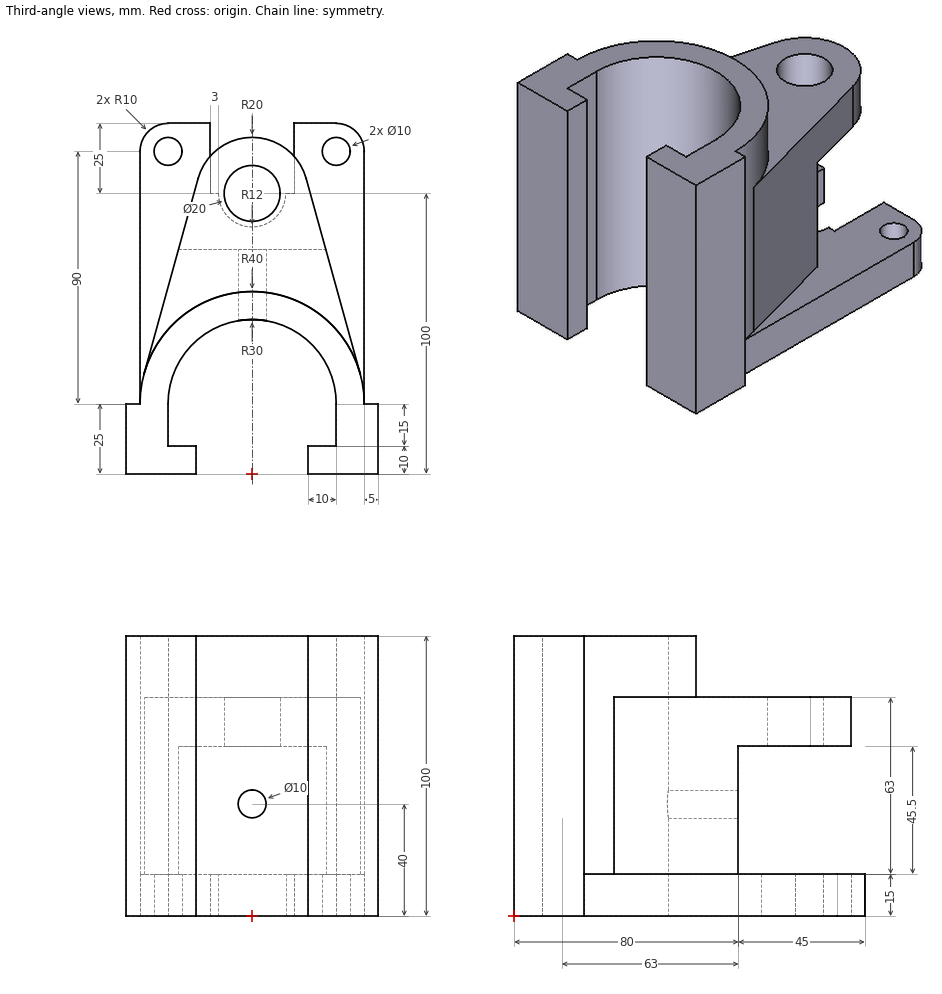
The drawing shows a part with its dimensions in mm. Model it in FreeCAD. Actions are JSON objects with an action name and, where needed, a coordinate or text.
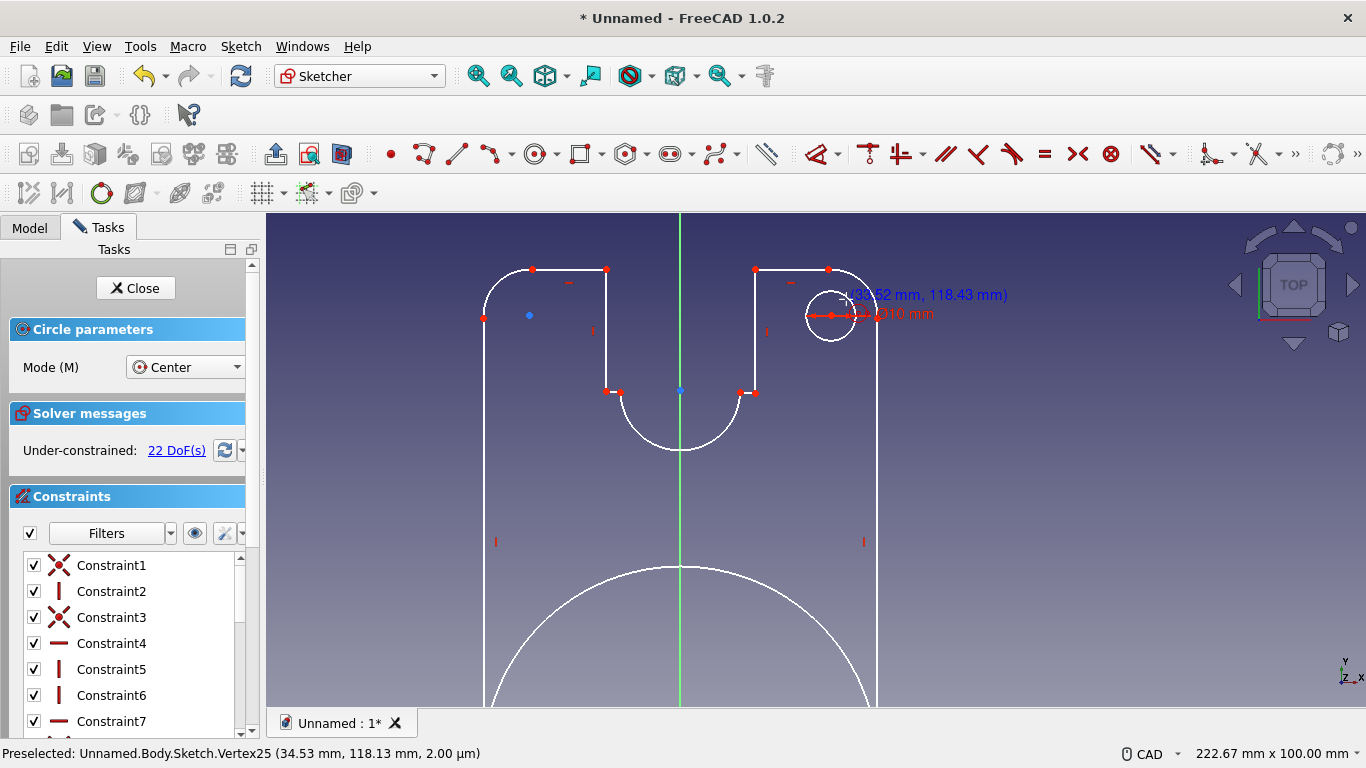
{"action": "left_click", "coordinate": [532, 317]}
{"action": "mouse_move", "coordinate": [550, 299]}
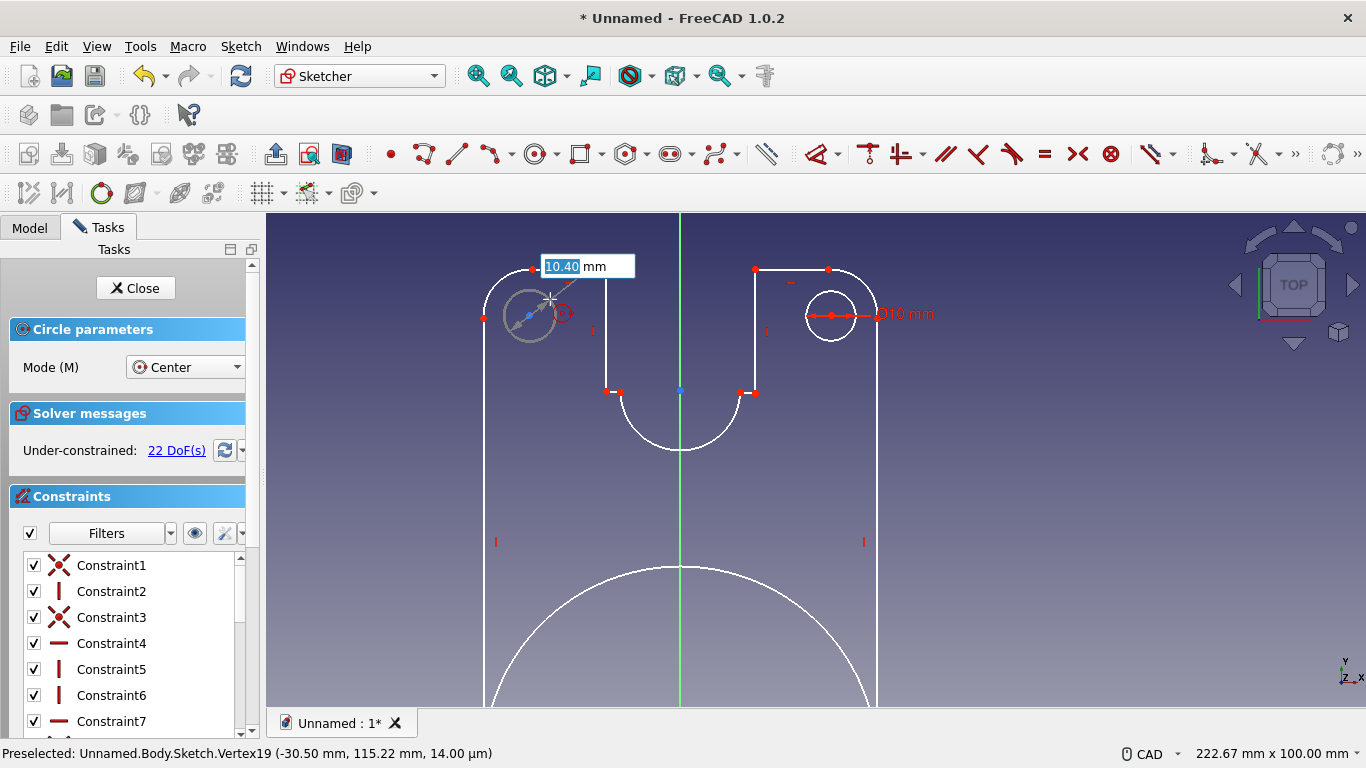
{"action": "type", "text": "10"}
{"action": "key", "text": "Return"}
{"action": "key", "text": "Escape"}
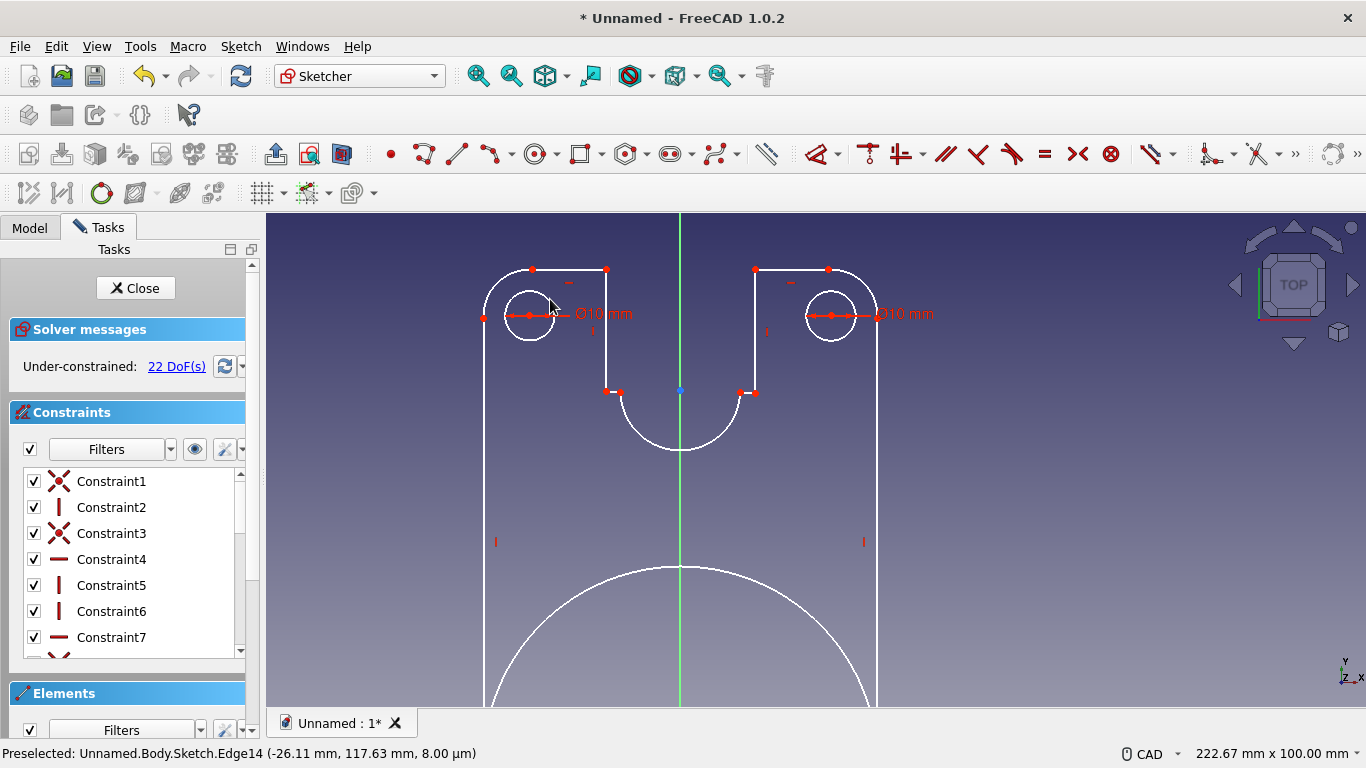
{"action": "left_click", "coordinate": [584, 270]}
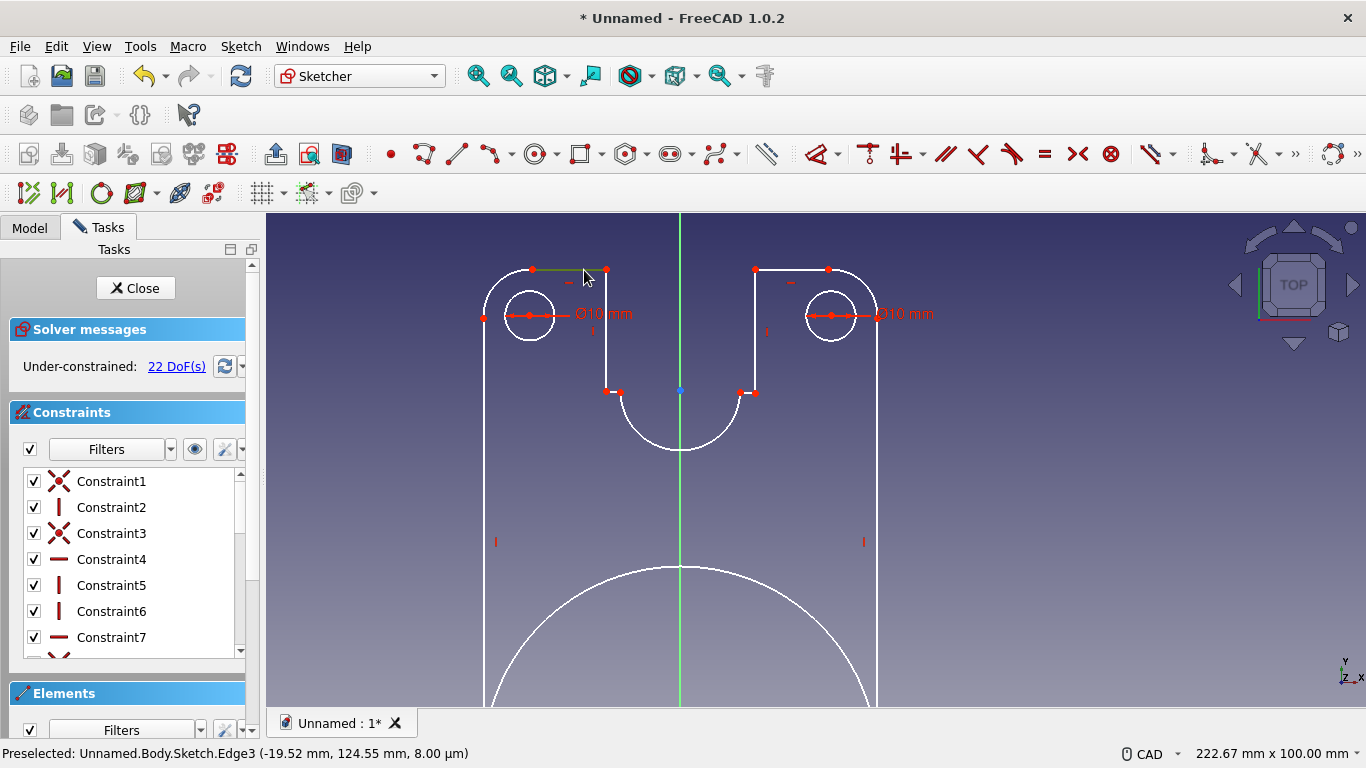
{"action": "left_click", "coordinate": [510, 274]}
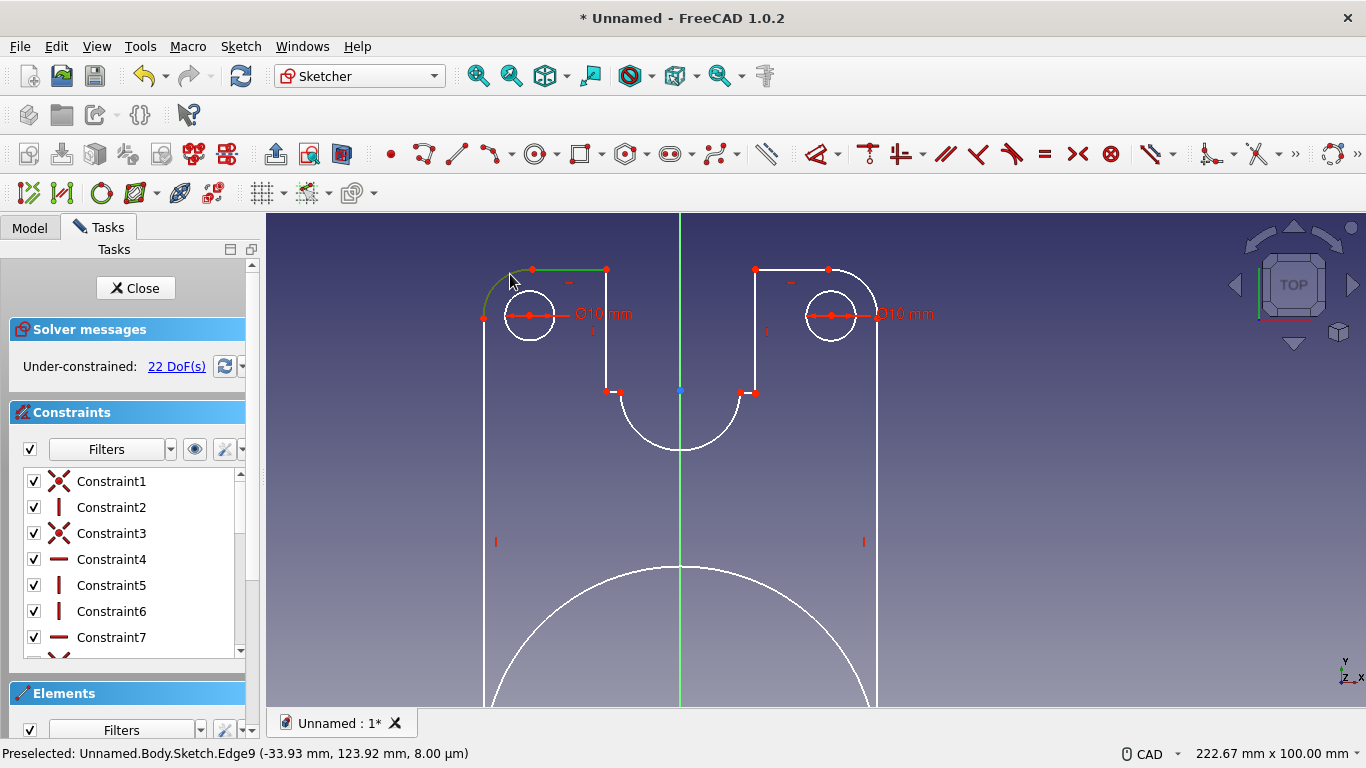
{"action": "key", "text": "t"}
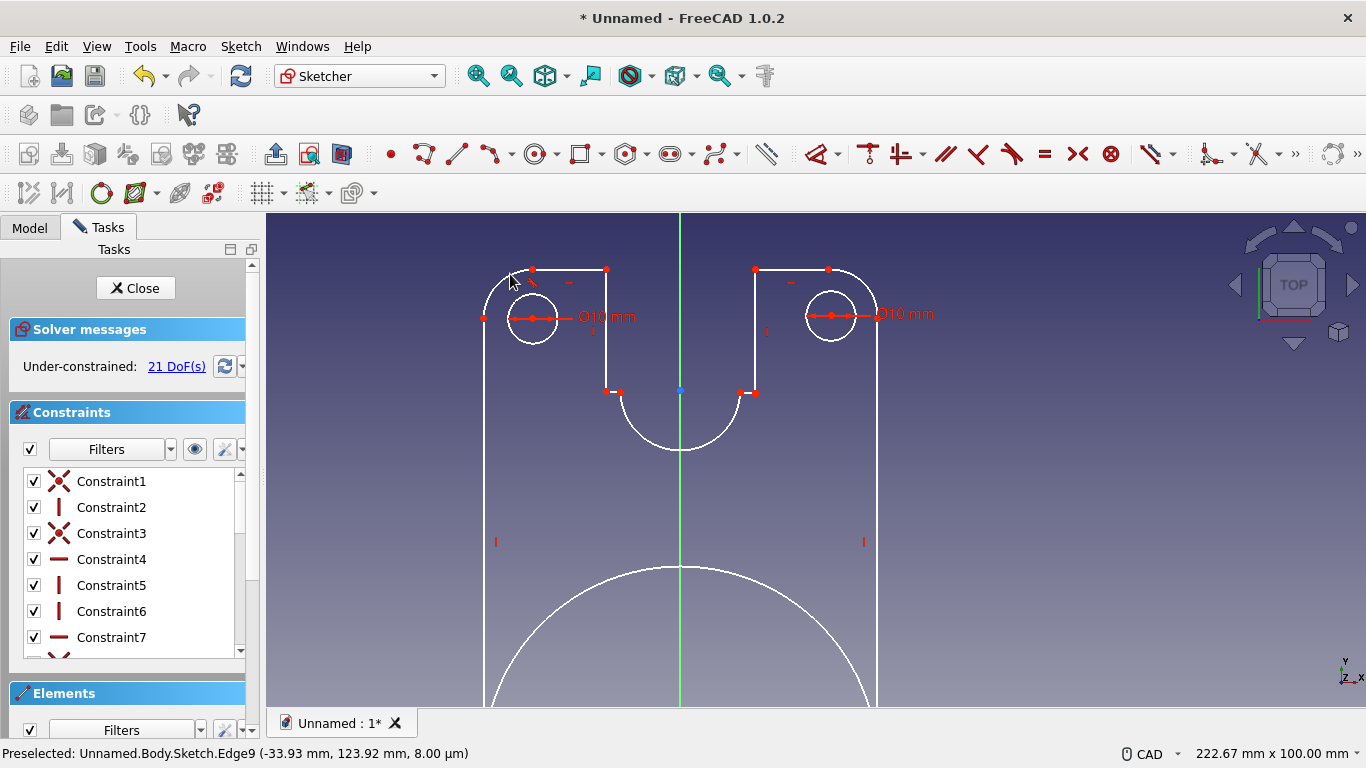
{"action": "left_click", "coordinate": [484, 452]}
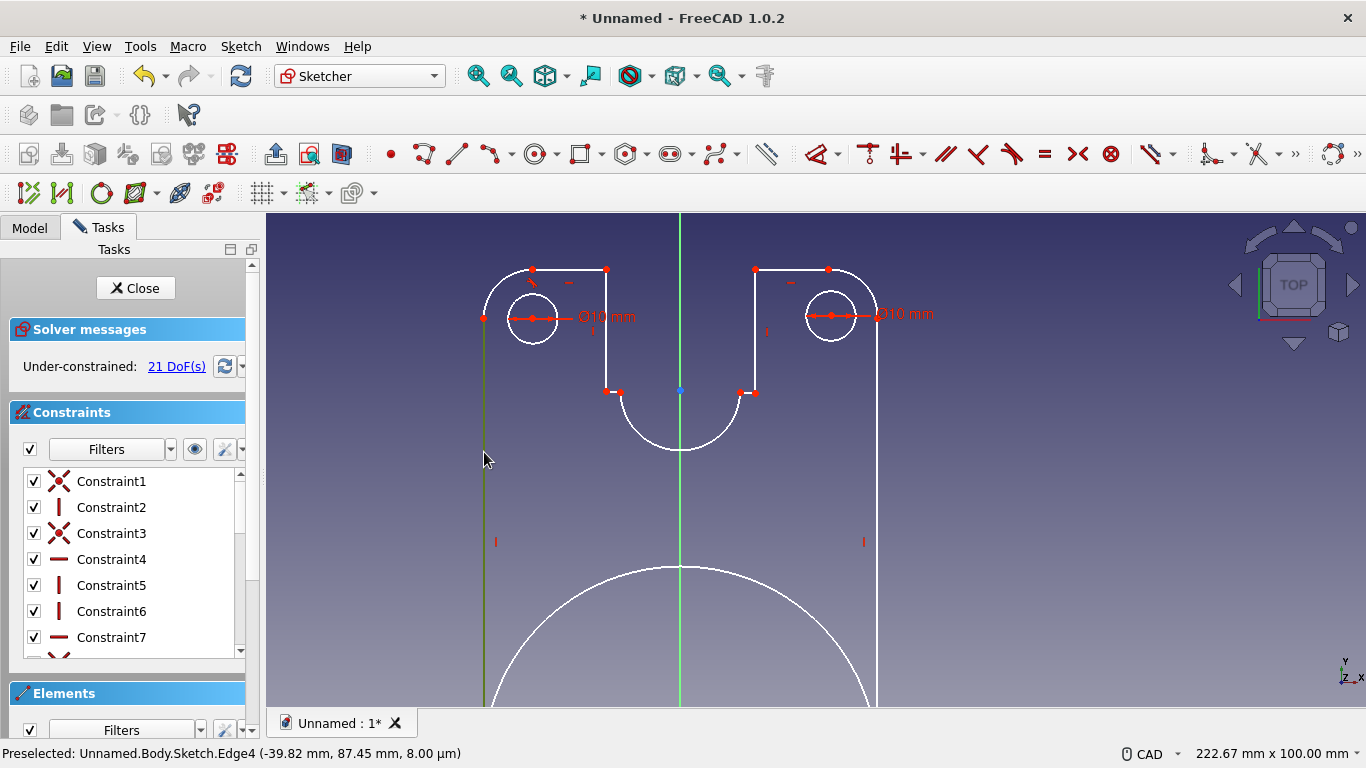
{"action": "left_click", "coordinate": [511, 275]}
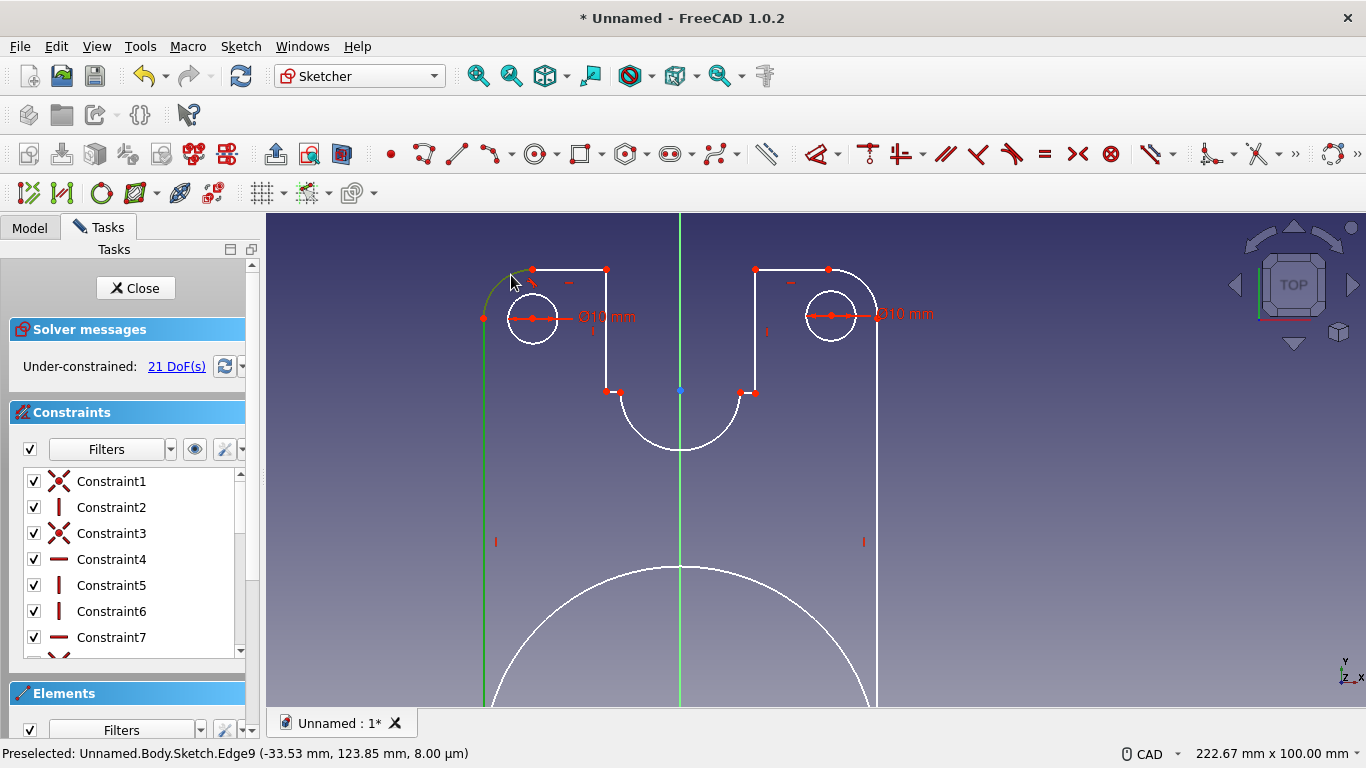
{"action": "key", "text": "t"}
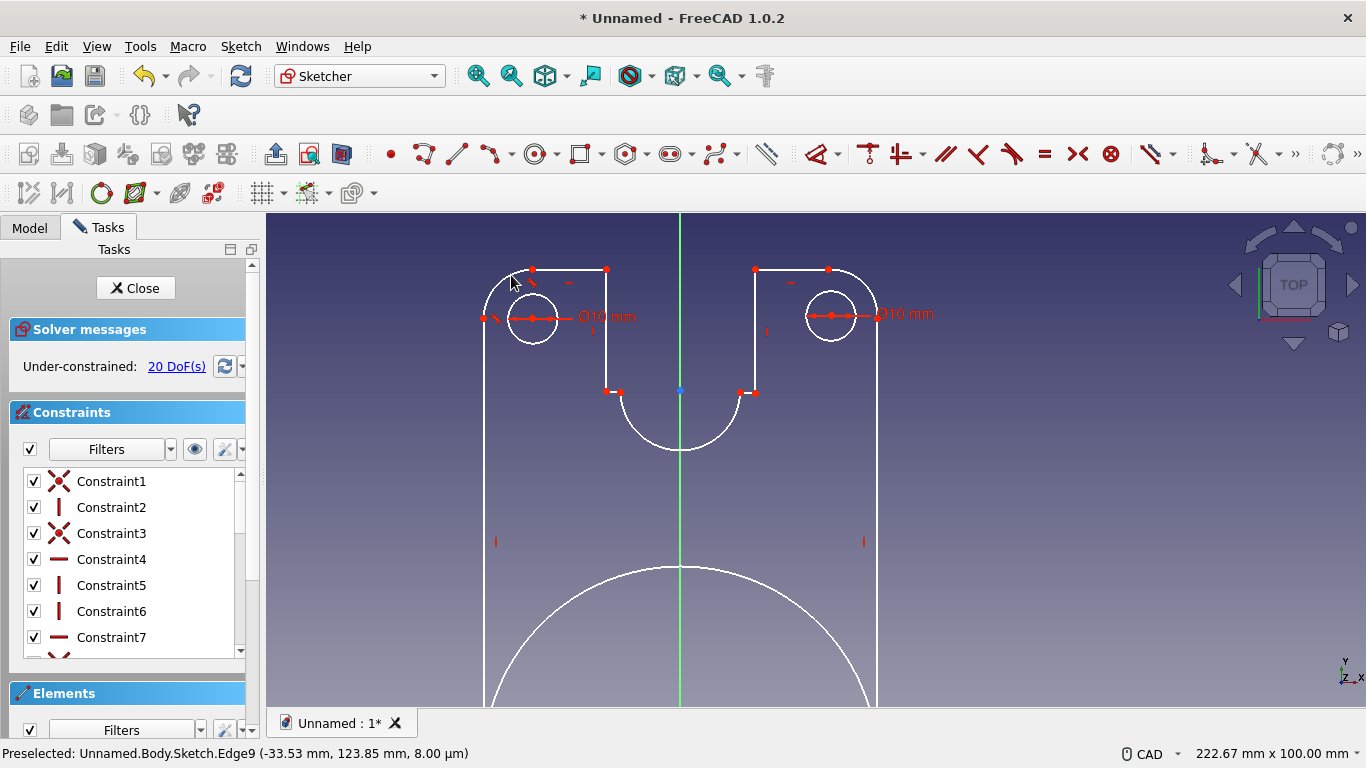
{"action": "left_click", "coordinate": [877, 630]}